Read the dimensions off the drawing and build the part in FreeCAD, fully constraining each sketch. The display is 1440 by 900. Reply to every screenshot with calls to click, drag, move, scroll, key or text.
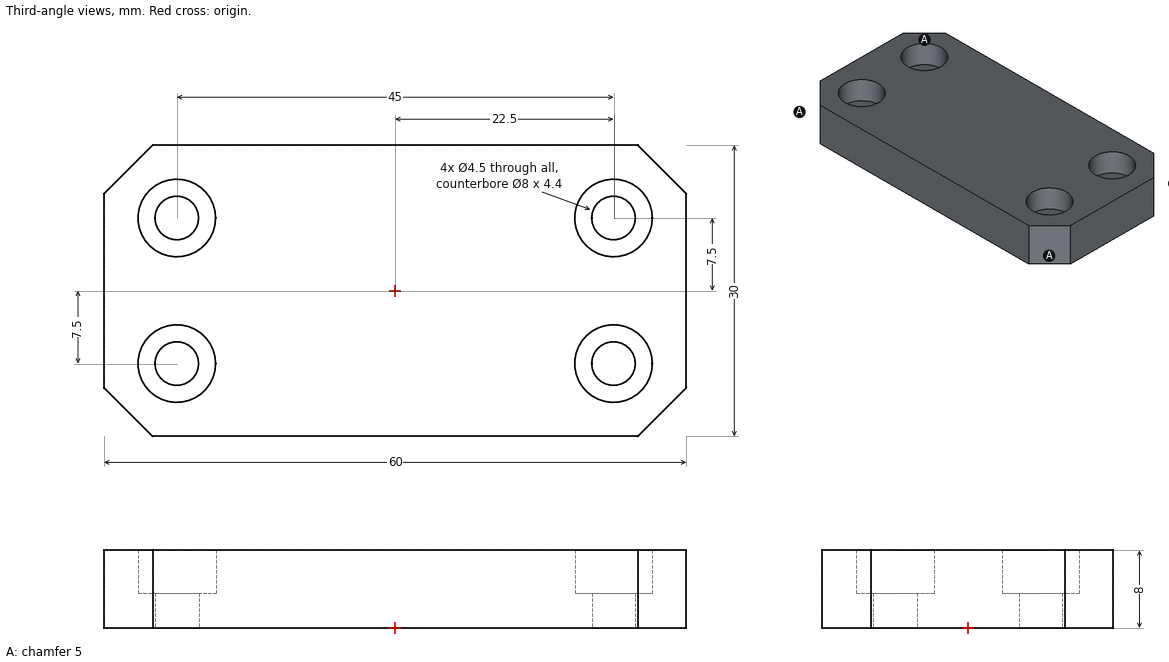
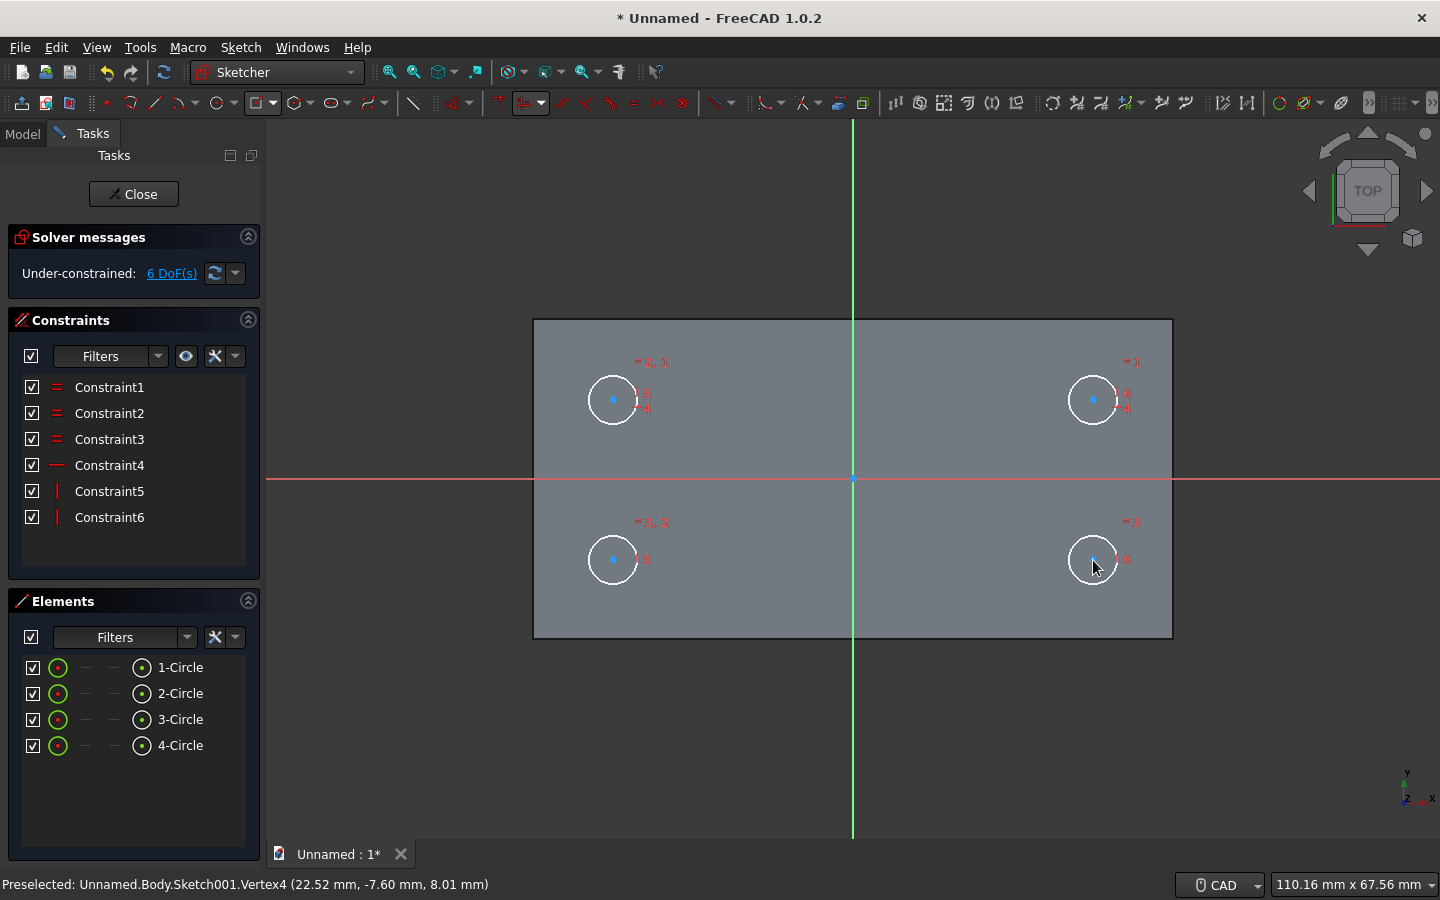
click(613, 560)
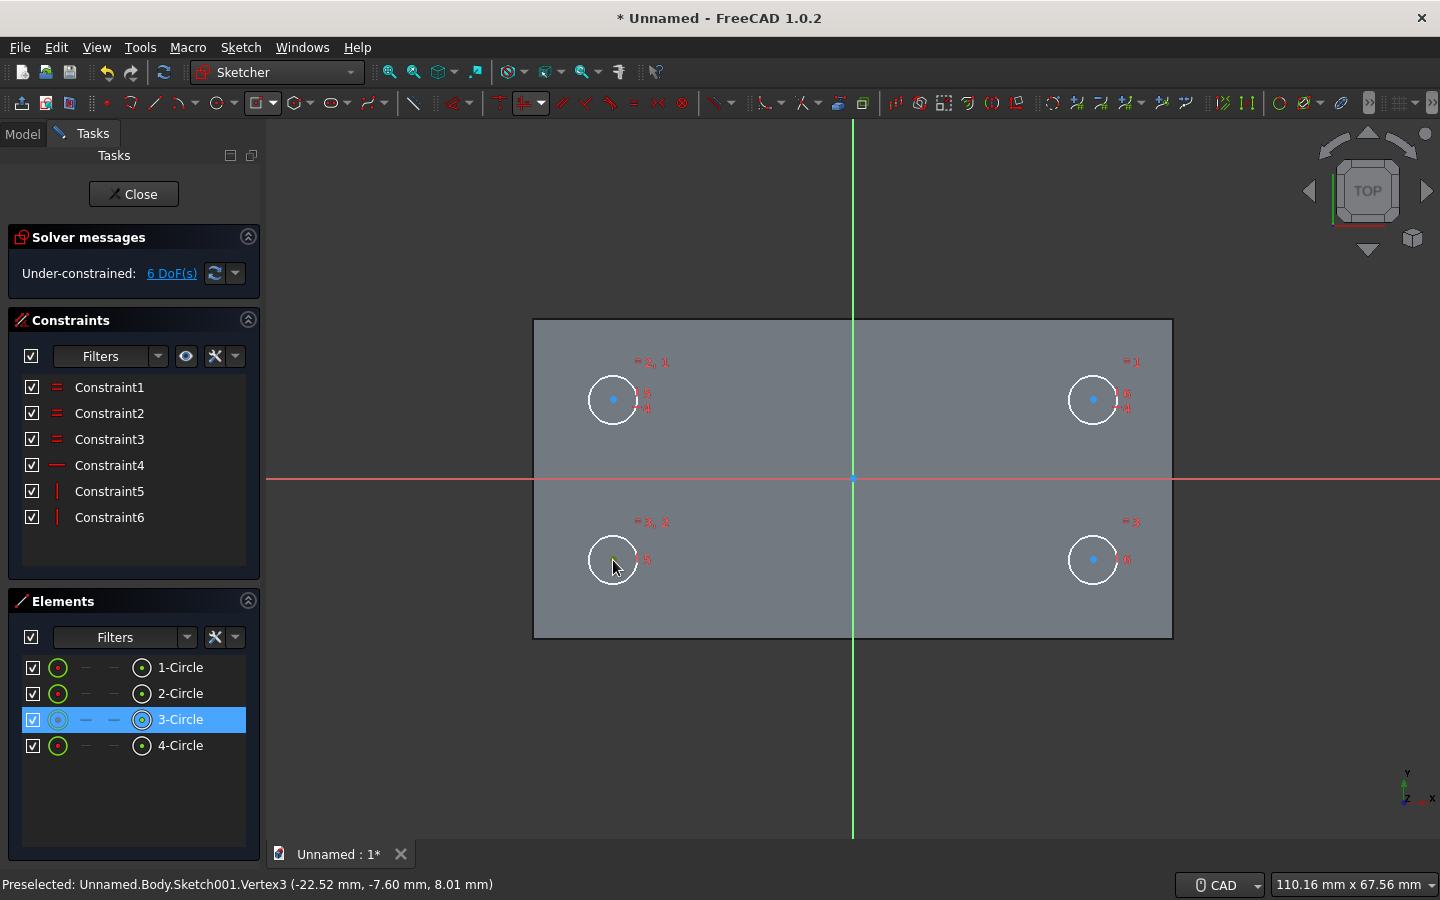
click(1093, 560)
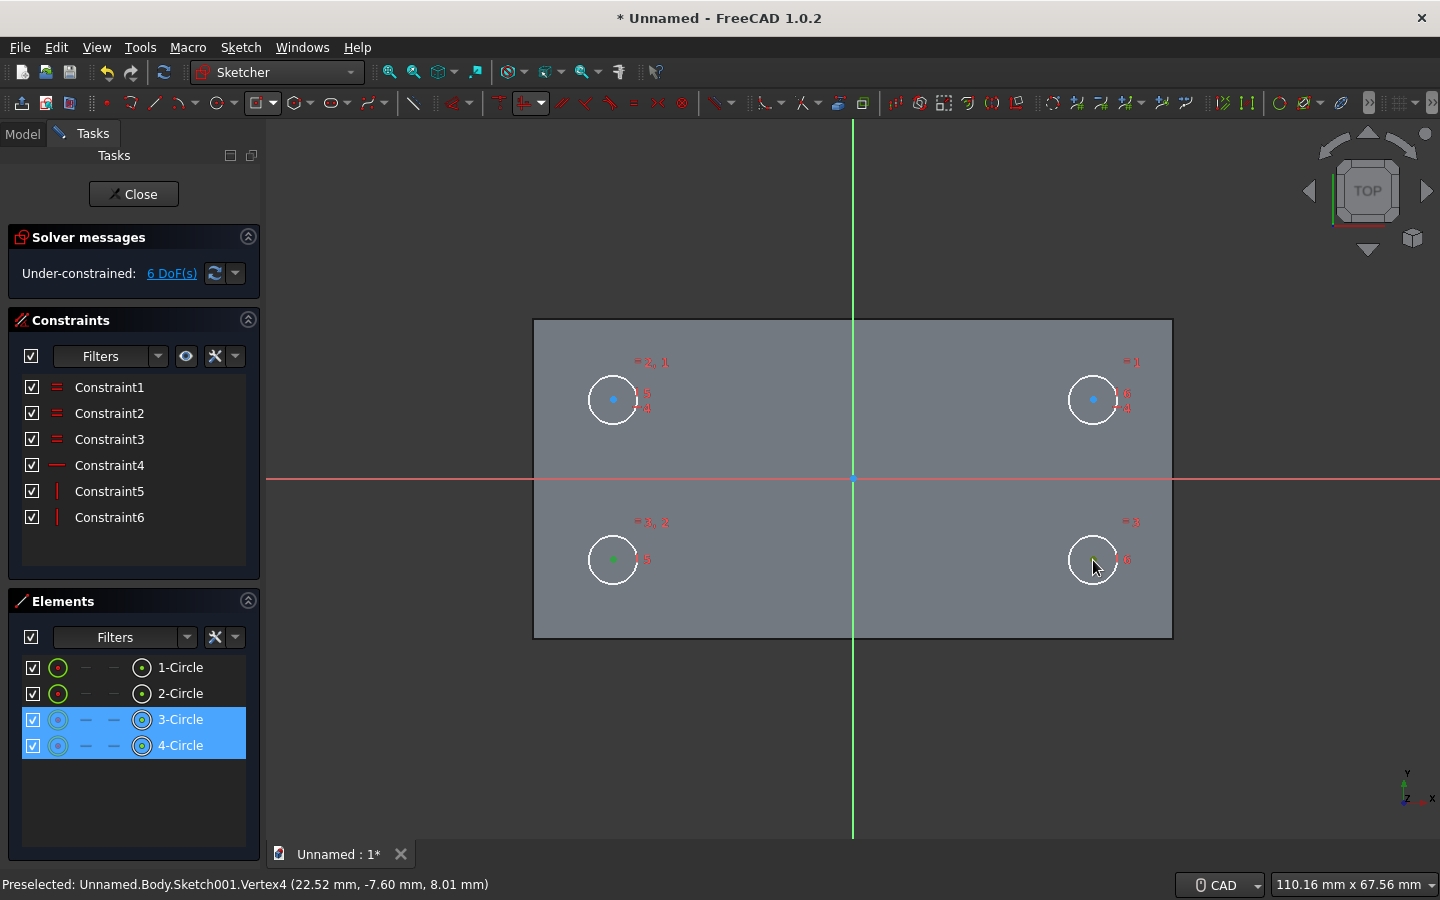
click(544, 104)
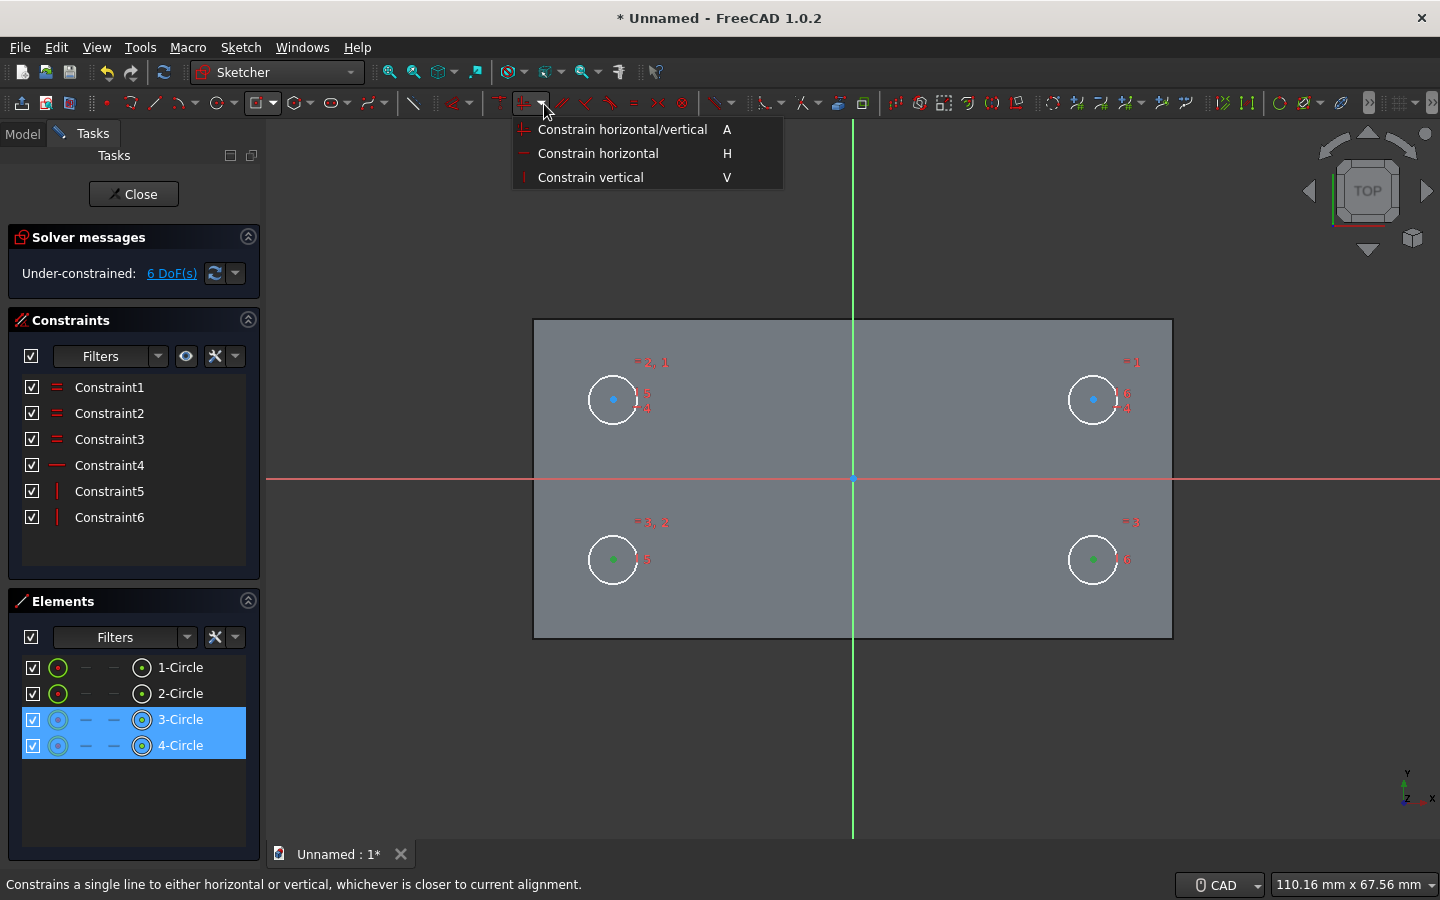
click(648, 153)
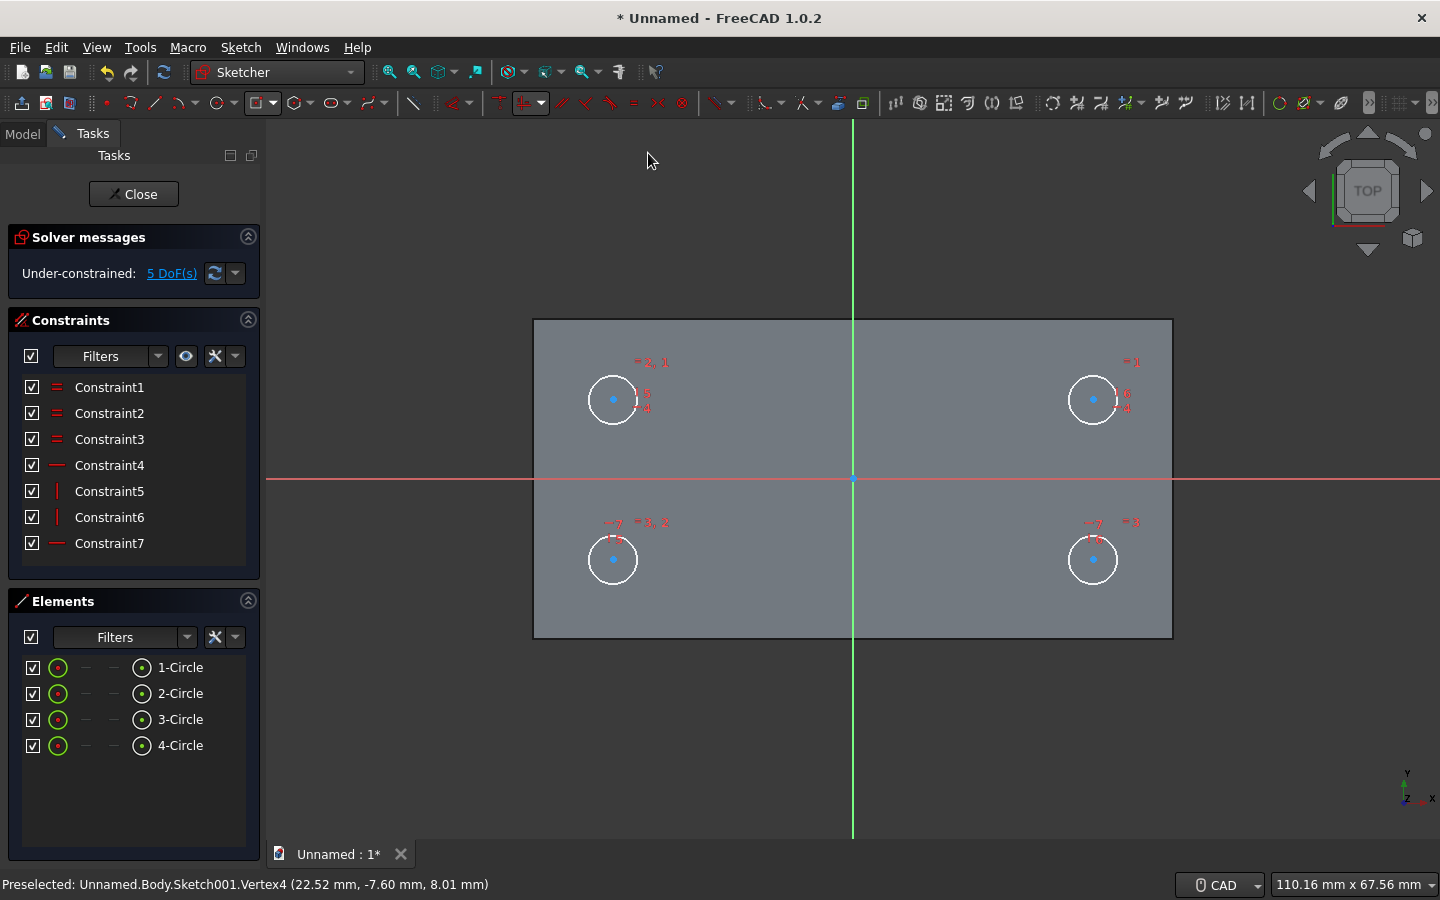
click(452, 104)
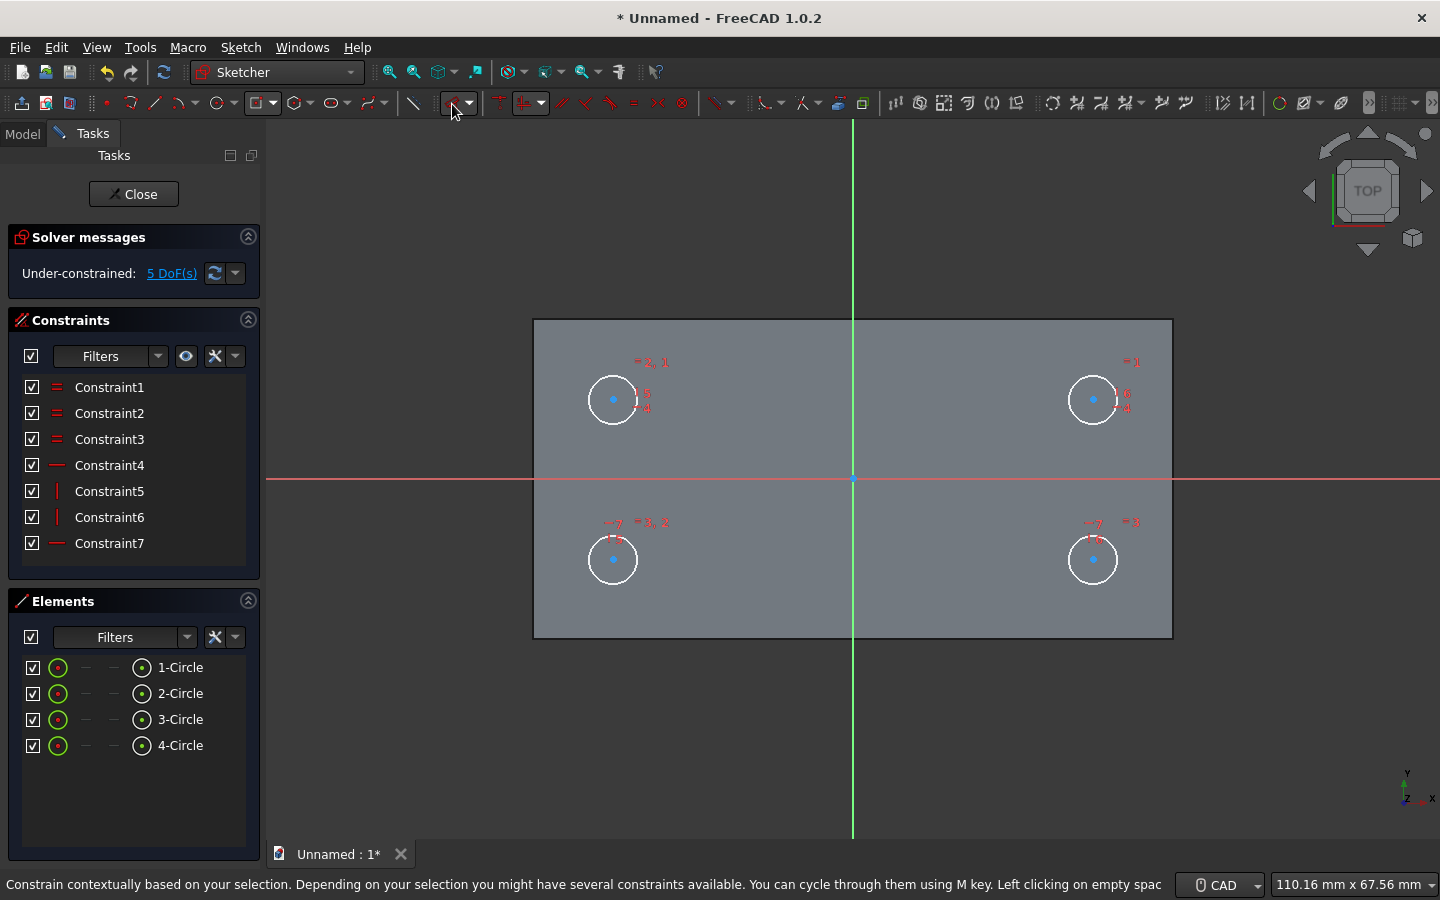
click(1110, 383)
click(1133, 360)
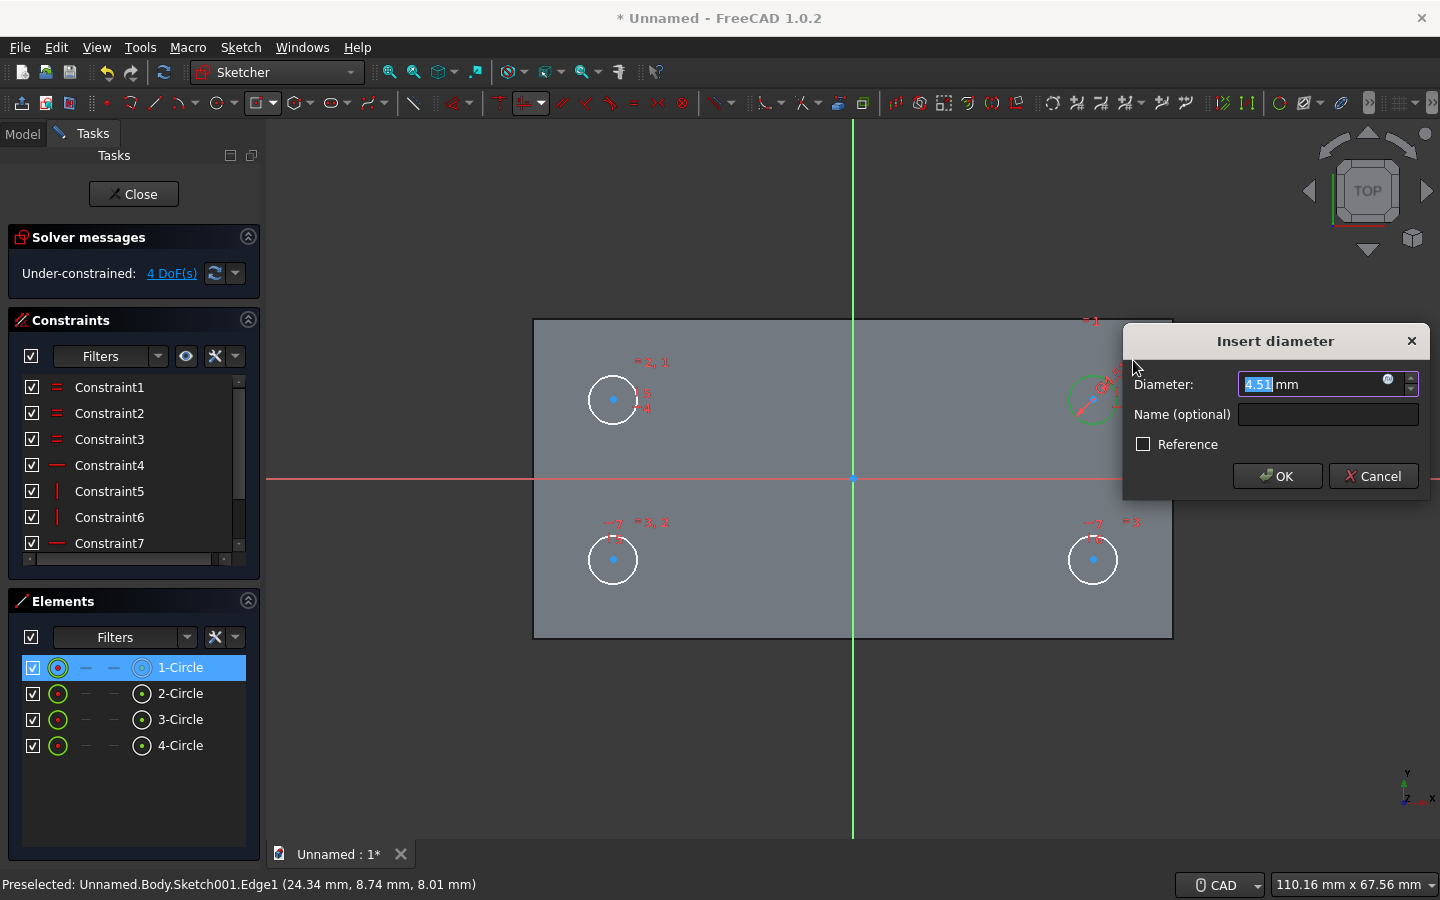
text(4.5)
key(Return)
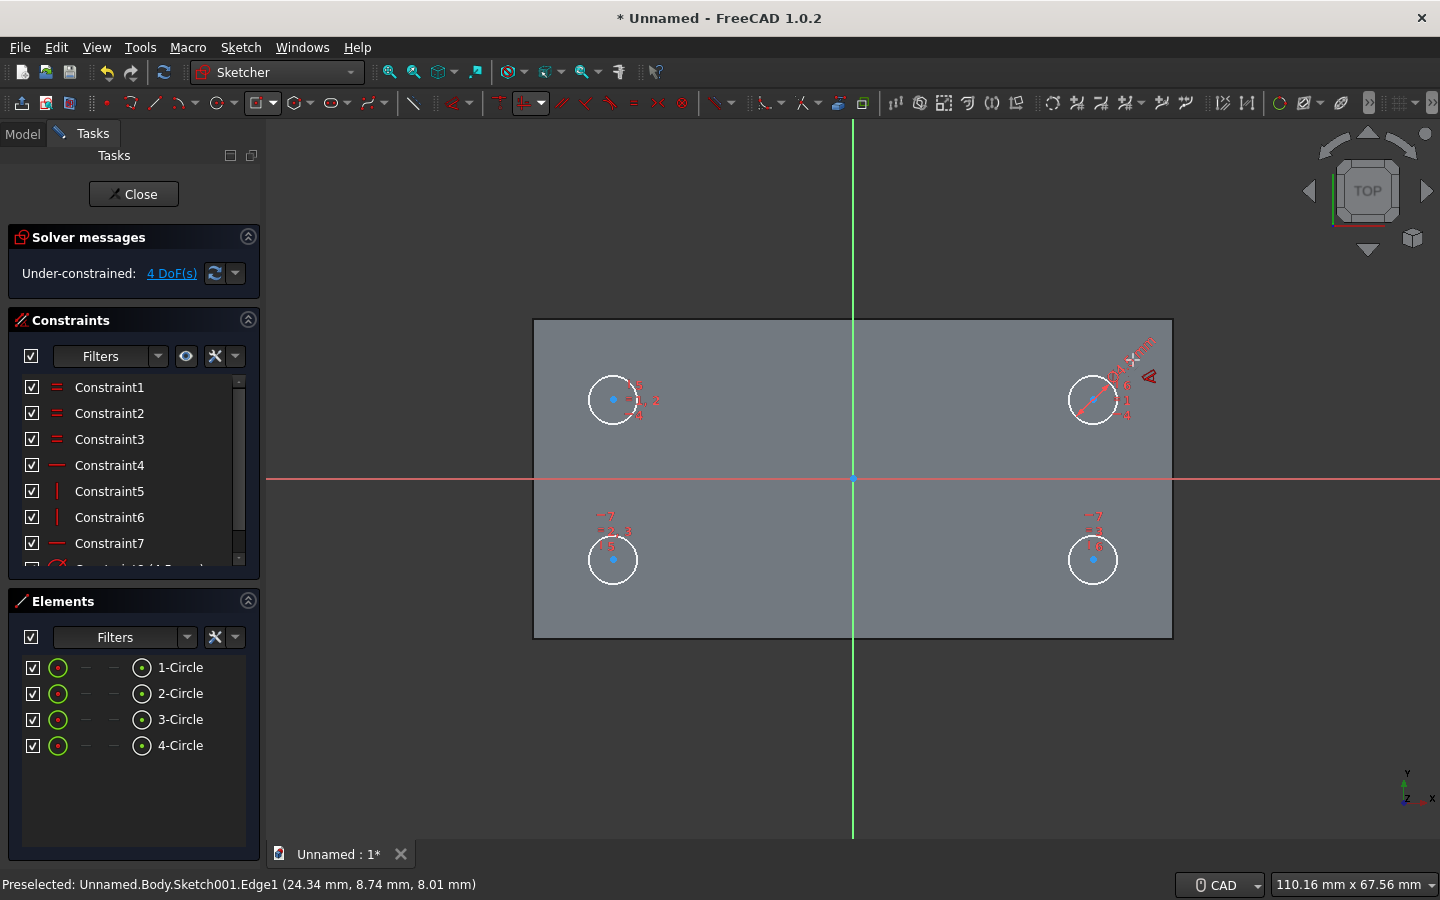
click(1093, 400)
click(1127, 440)